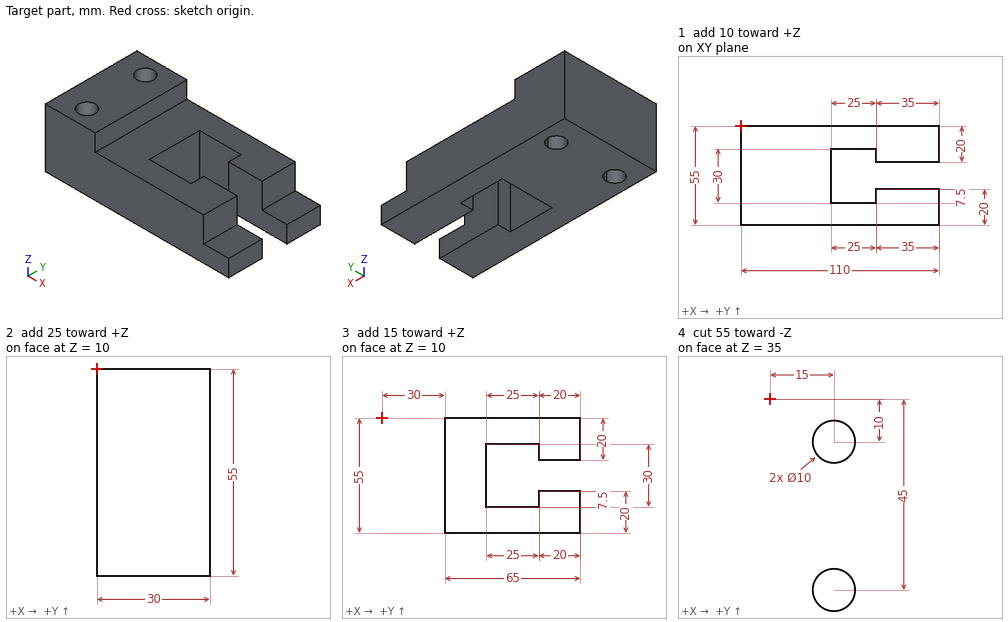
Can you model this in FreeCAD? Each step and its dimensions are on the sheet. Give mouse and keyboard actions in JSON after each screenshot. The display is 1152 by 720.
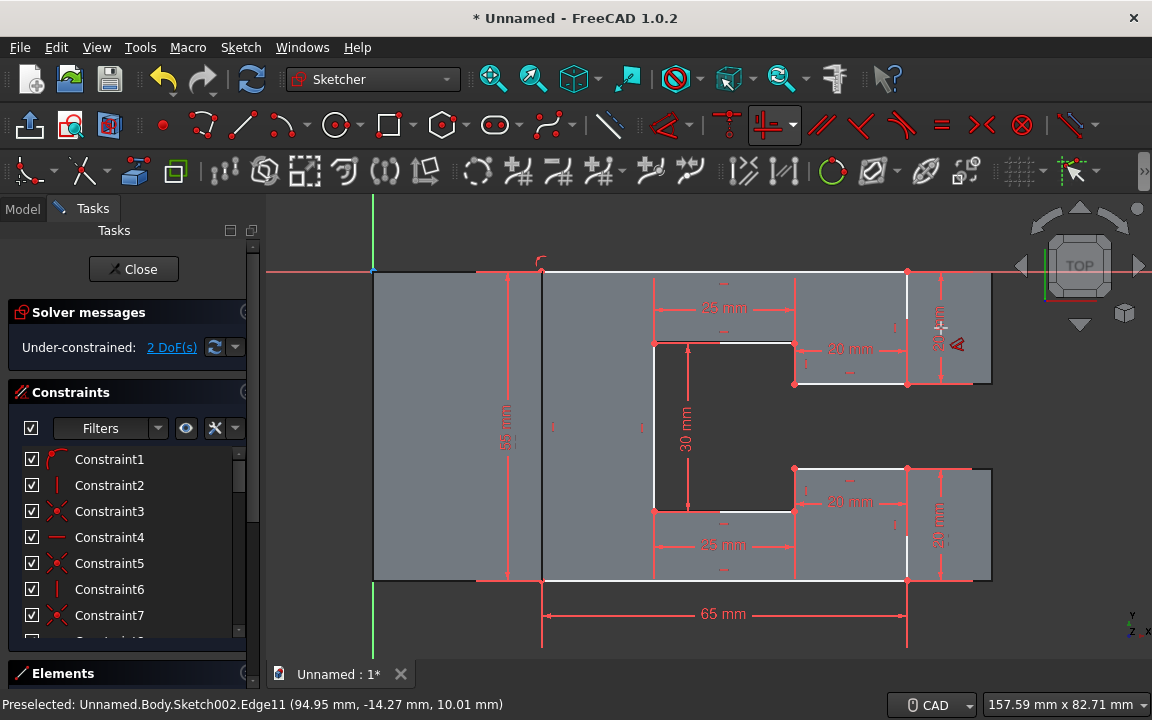
{"action": "left_click", "coordinate": [795, 482]}
{"action": "left_click", "coordinate": [761, 490]}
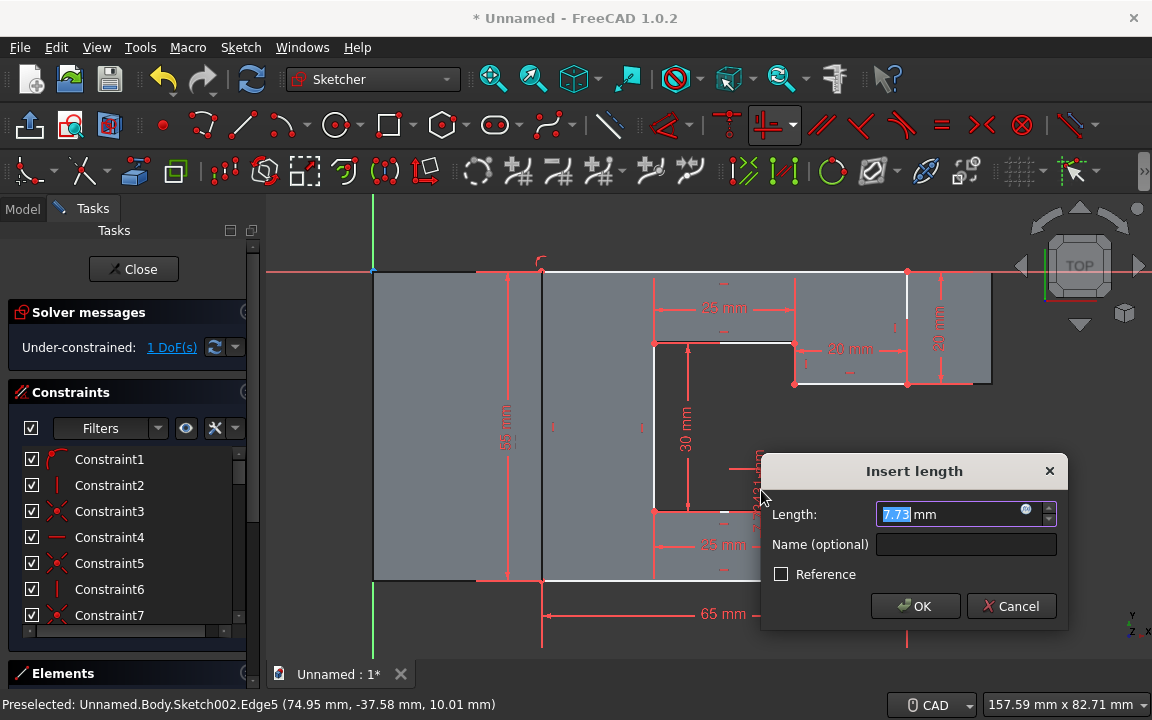
{"action": "type", "text": "7.5"}
{"action": "key", "text": "Return"}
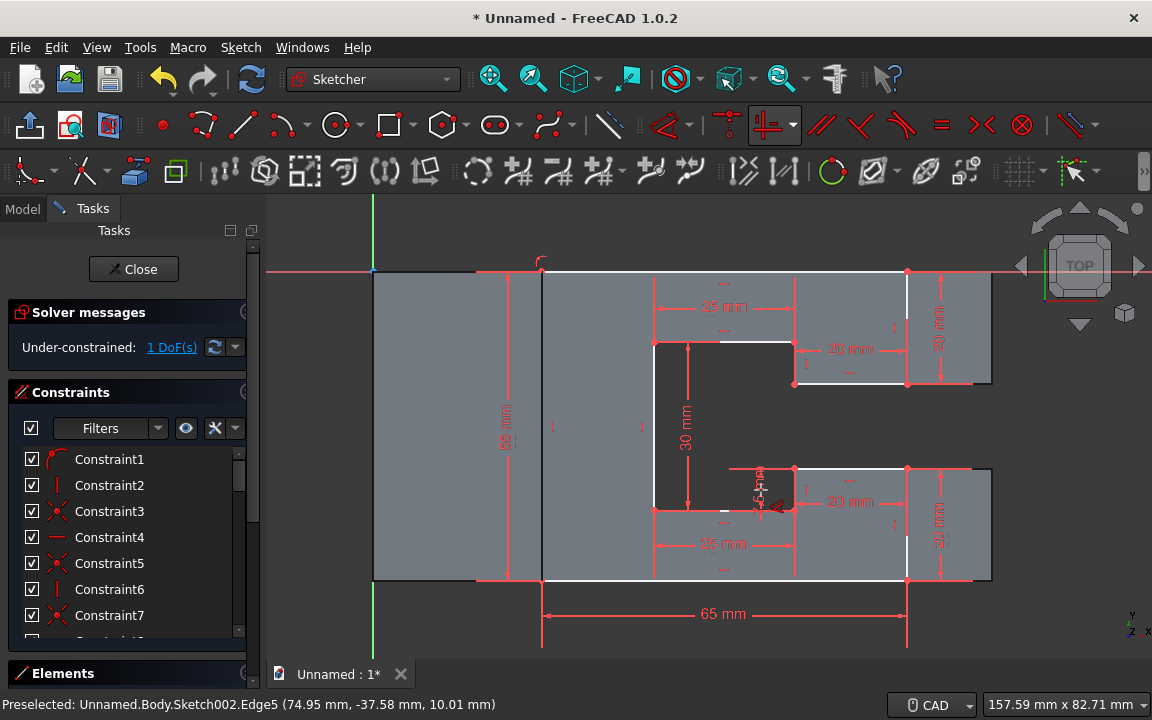
{"action": "left_click", "coordinate": [542, 272]}
{"action": "left_click", "coordinate": [457, 238]}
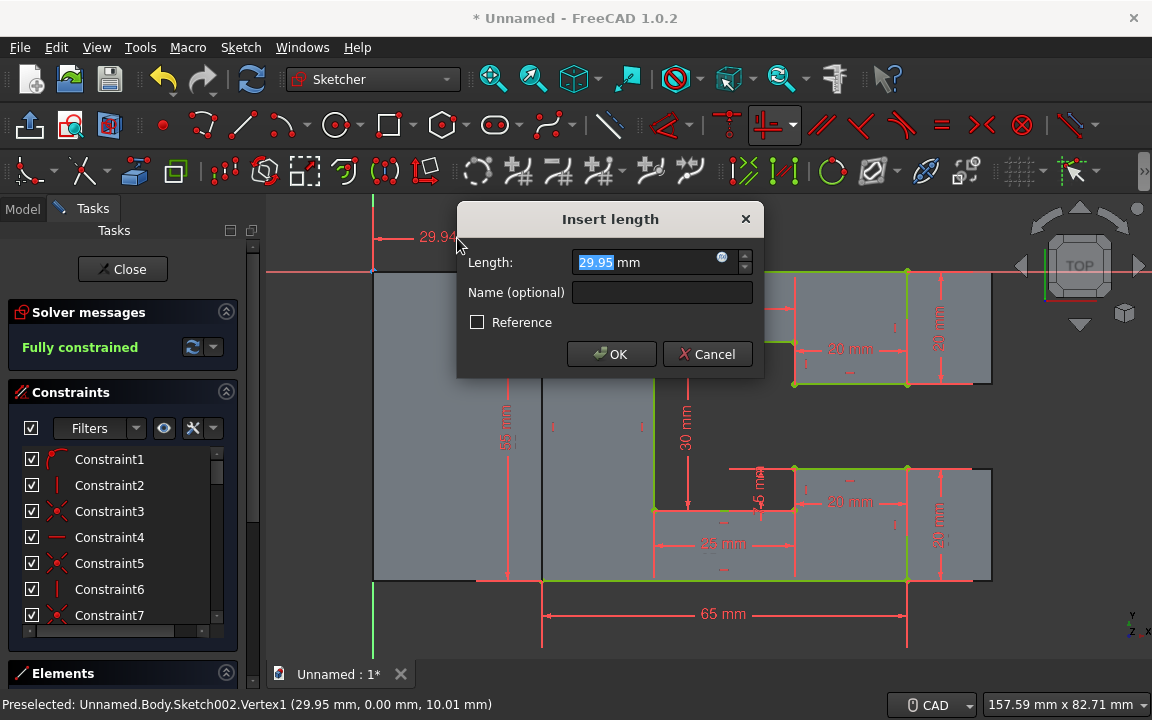
{"action": "type", "text": "30"}
{"action": "key", "text": "Return"}
{"action": "key", "text": "Escape"}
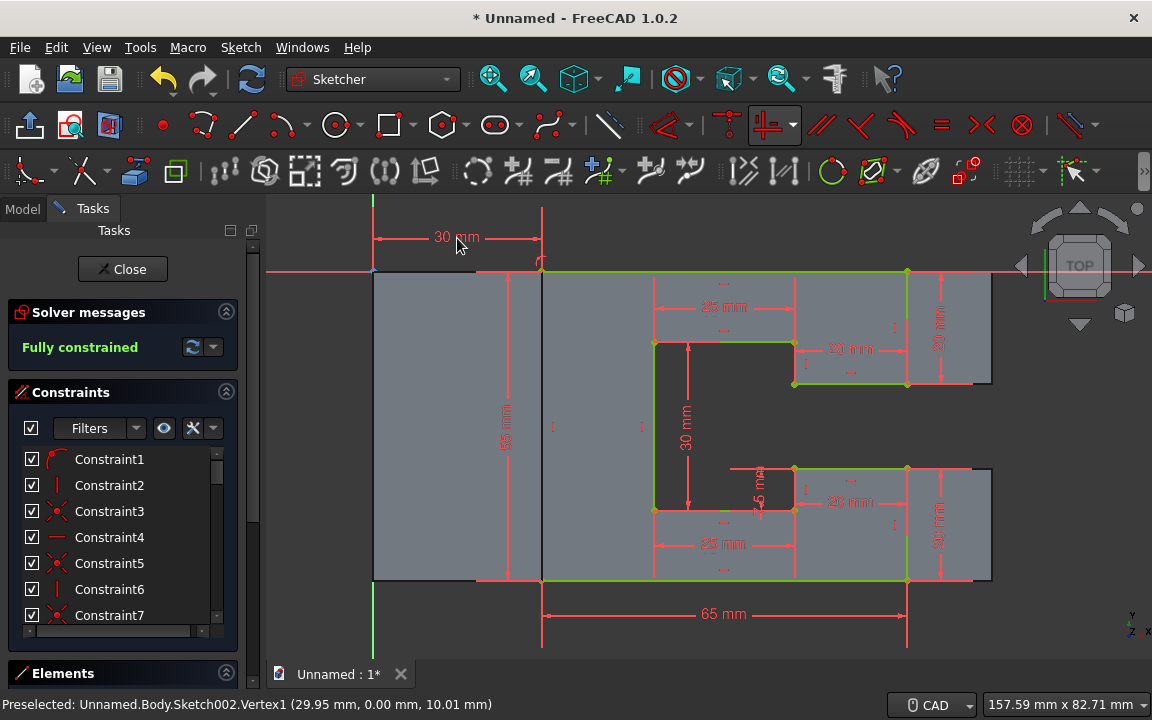
{"action": "left_click", "coordinate": [123, 269]}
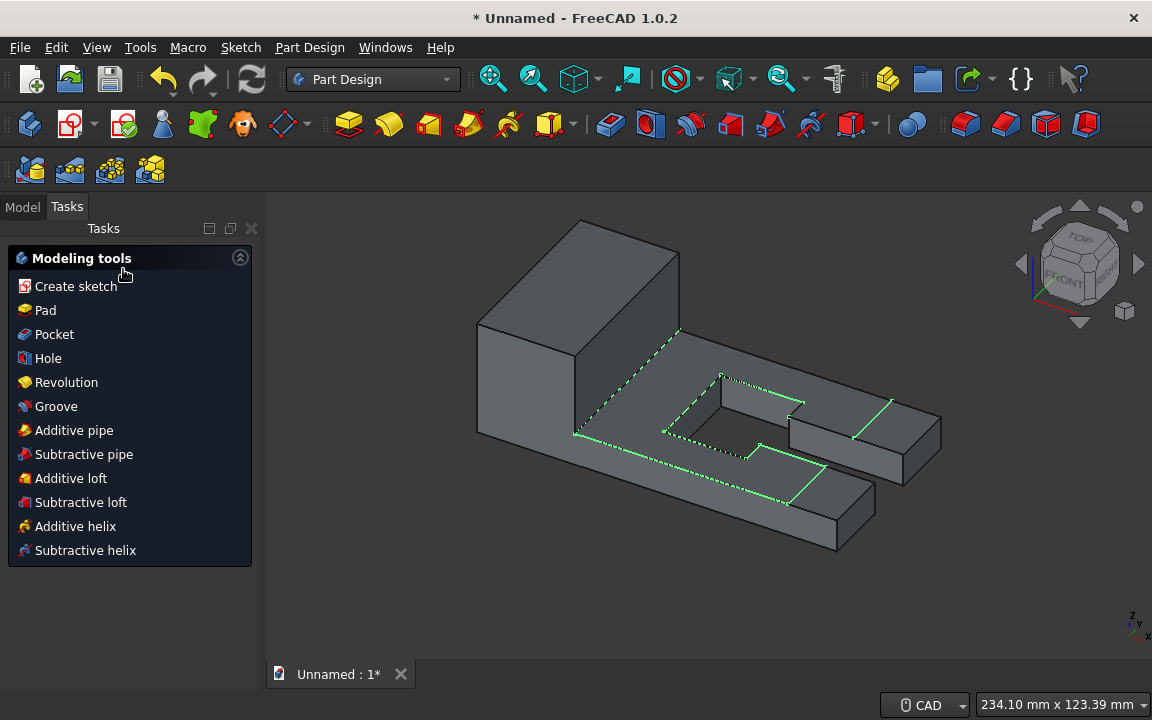
{"action": "left_click", "coordinate": [350, 124]}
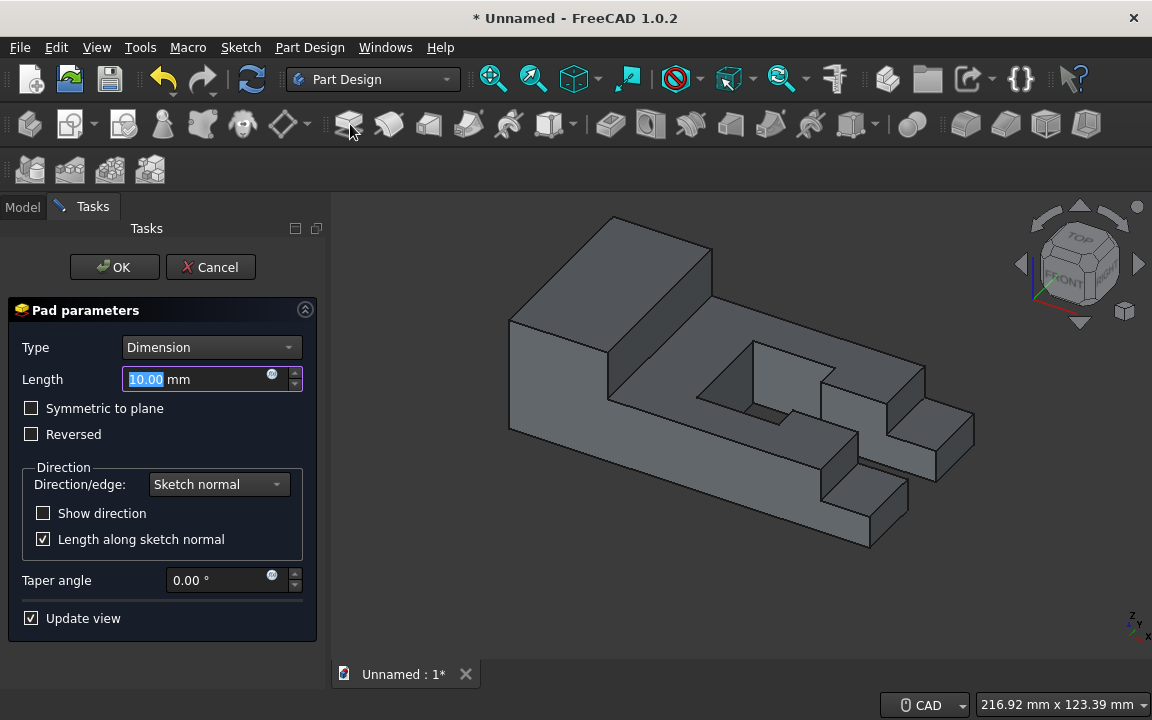
{"action": "type", "text": "15"}
{"action": "key", "text": "Tab"}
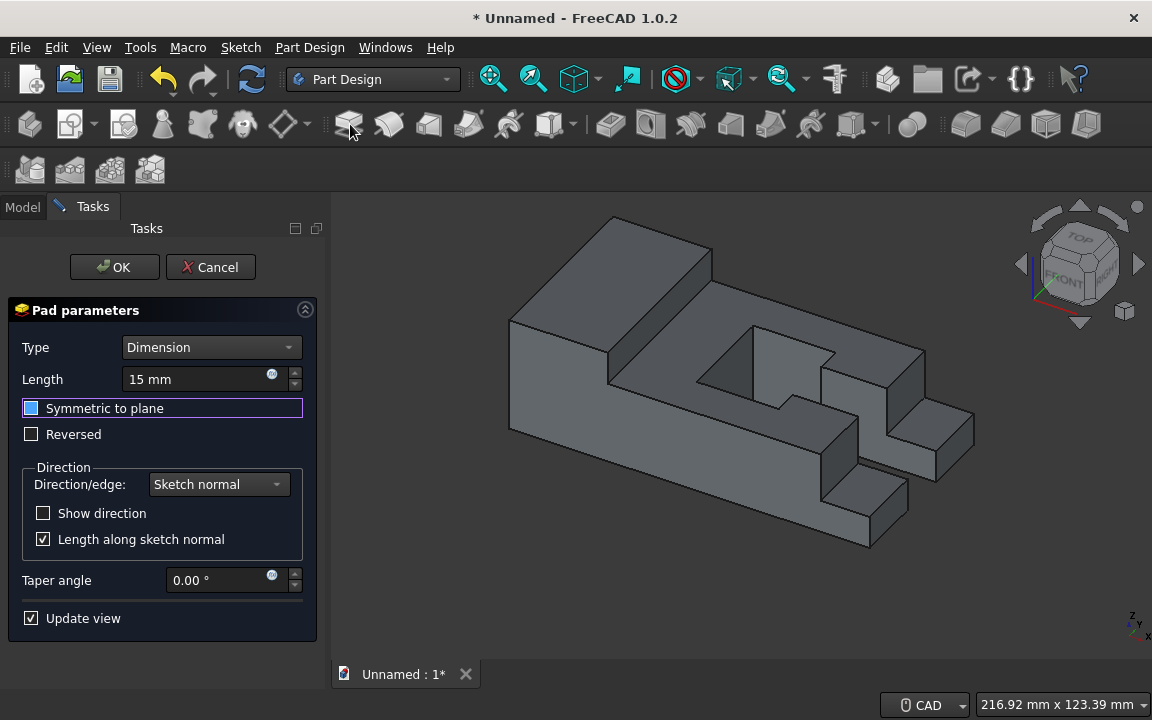
{"action": "left_click", "coordinate": [115, 267]}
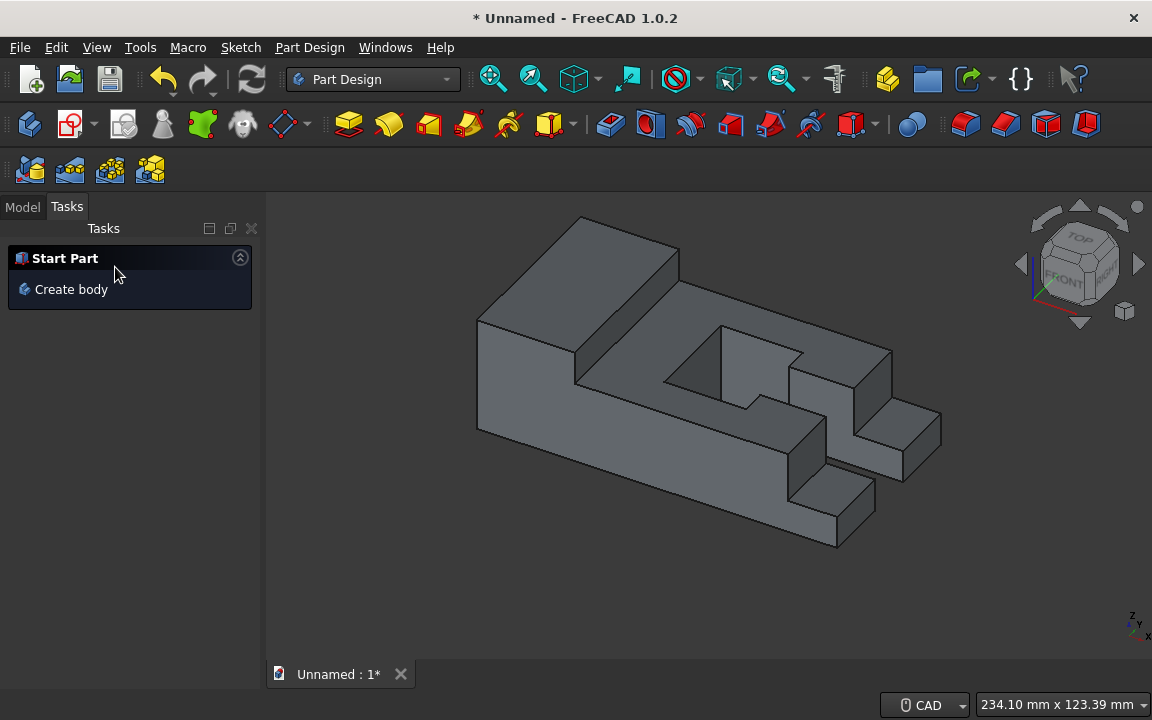
{"action": "left_click", "coordinate": [593, 269]}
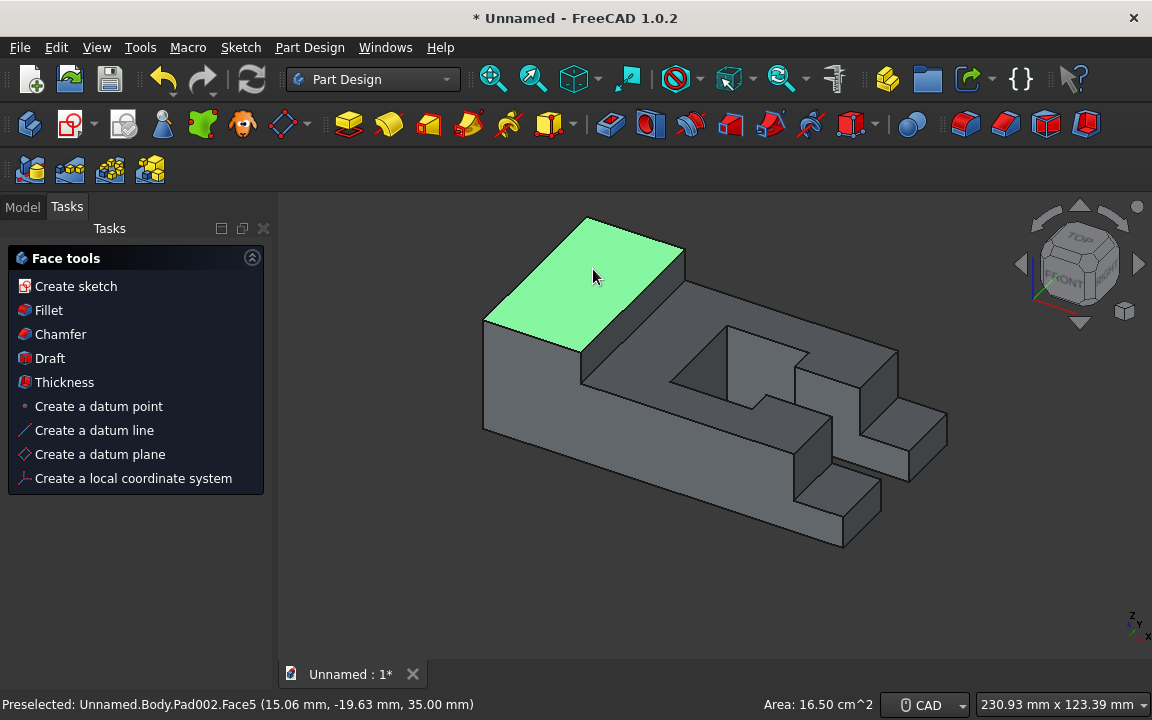
{"action": "left_click", "coordinate": [70, 124]}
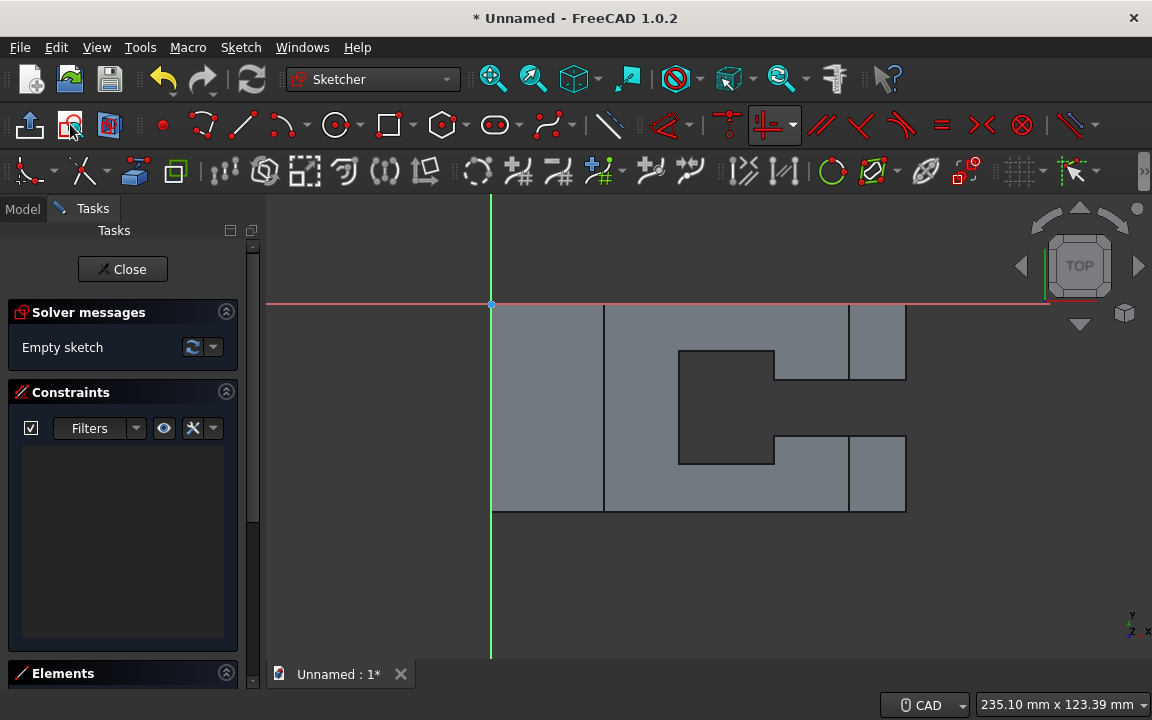
{"action": "scroll", "coordinate": [301, 342], "scroll_direction": "up", "scroll_amount": 2}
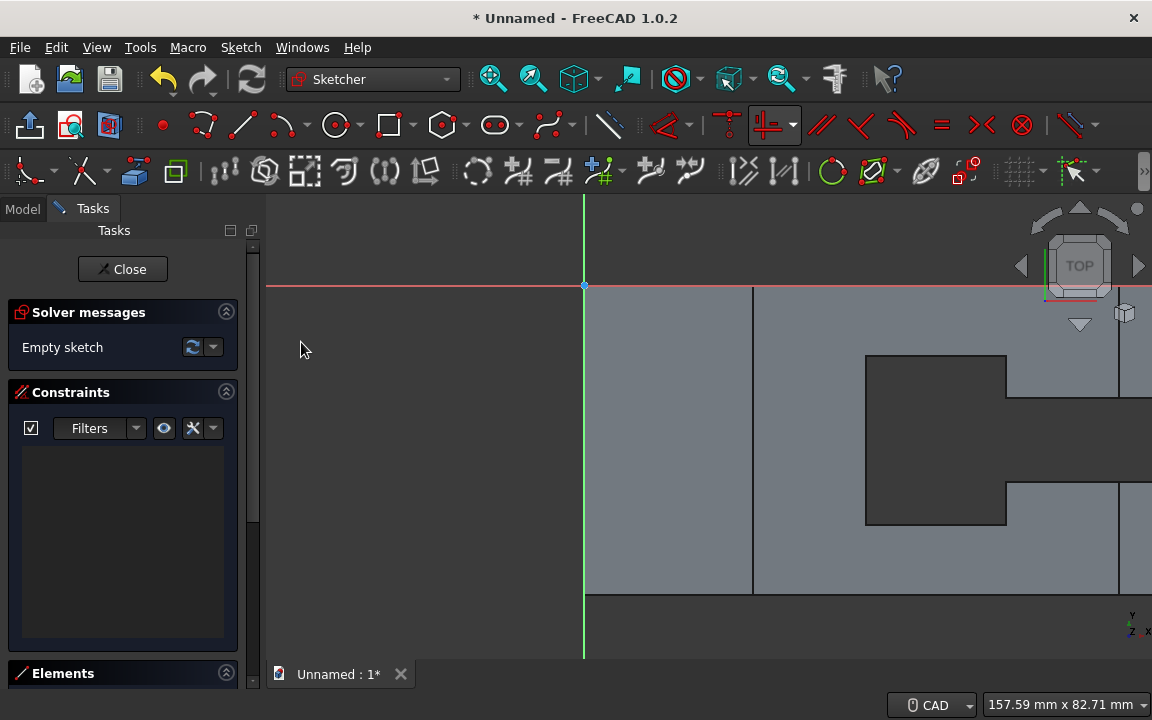
{"action": "left_click", "coordinate": [336, 126]}